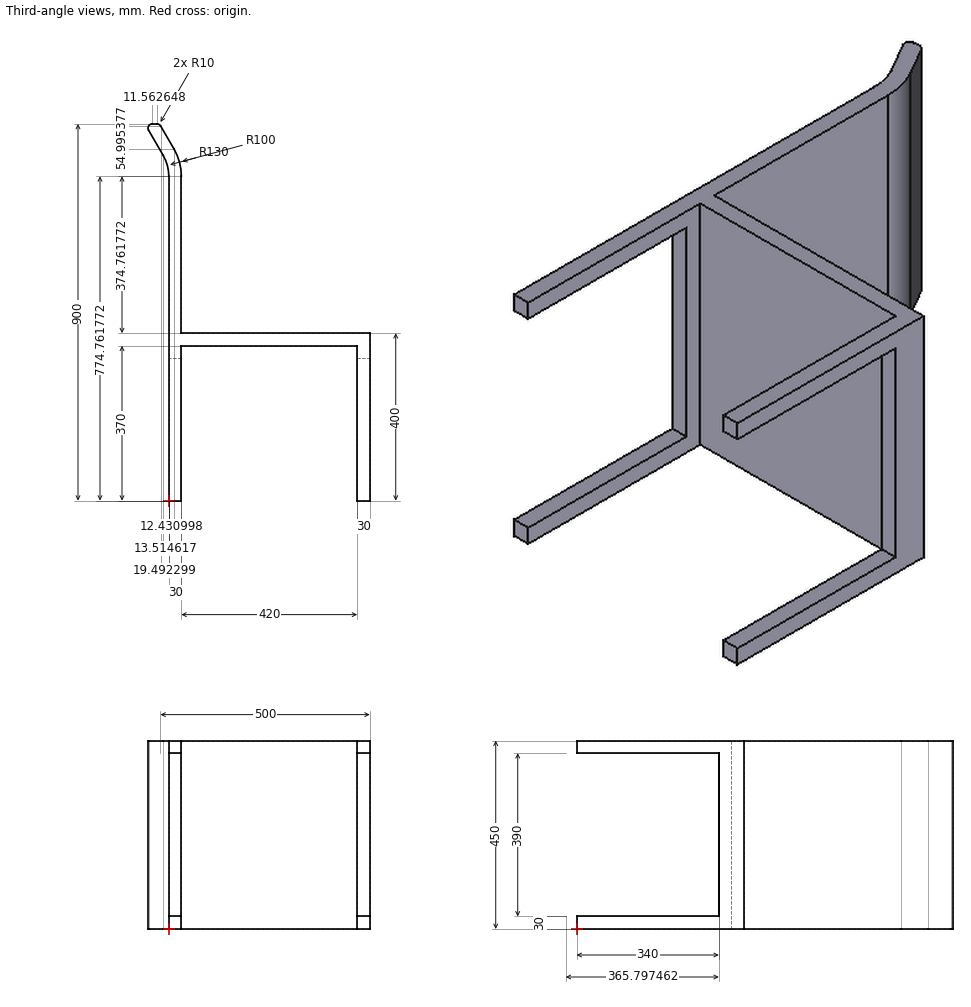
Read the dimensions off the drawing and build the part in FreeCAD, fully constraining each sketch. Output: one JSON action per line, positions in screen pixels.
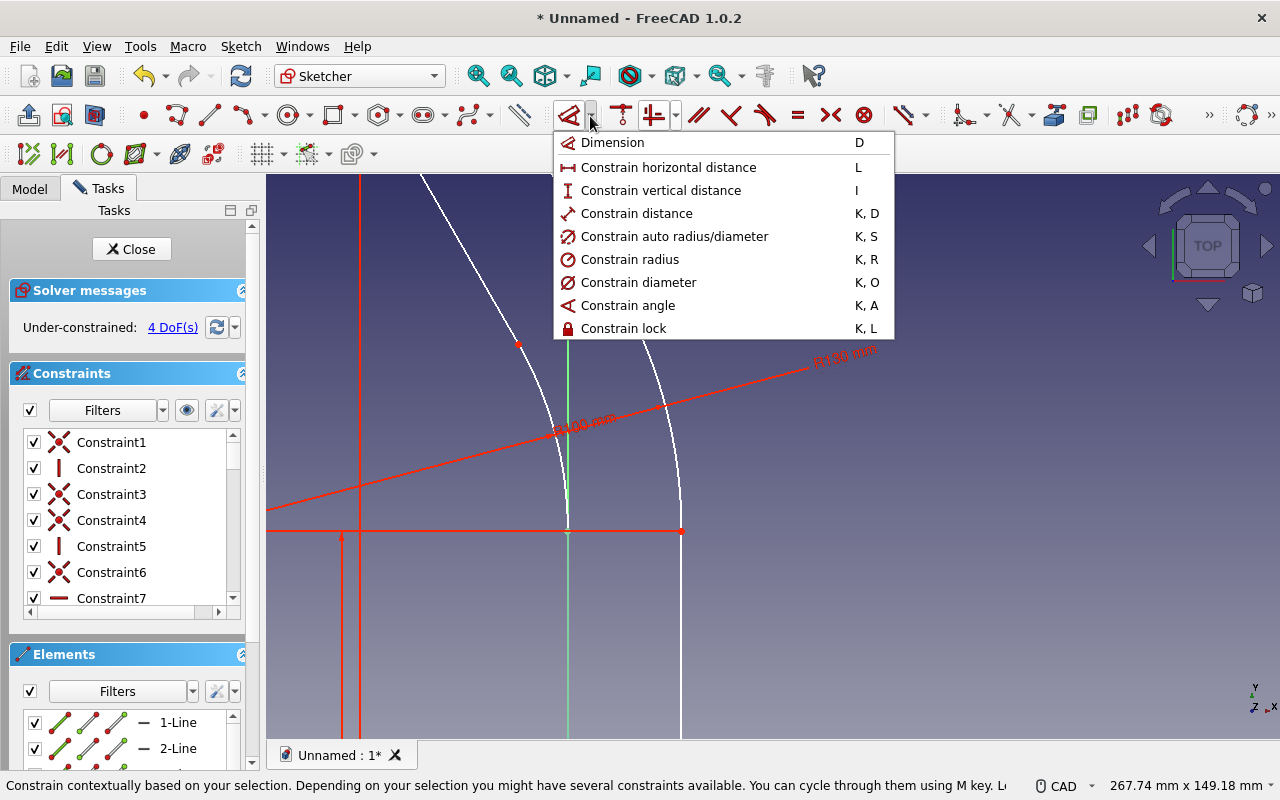
{"action": "left_click", "coordinate": [724, 168]}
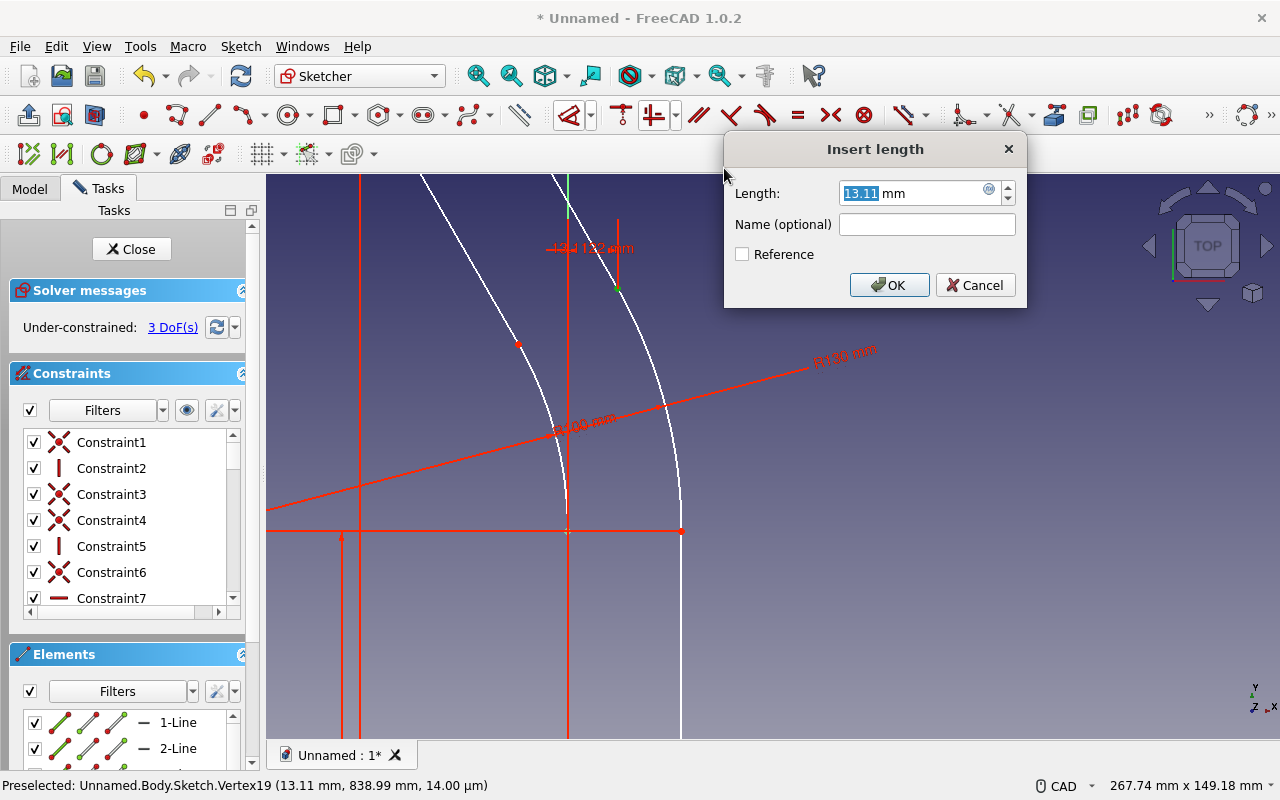
{"action": "type", "text": "12.430998"}
{"action": "key", "text": "Return"}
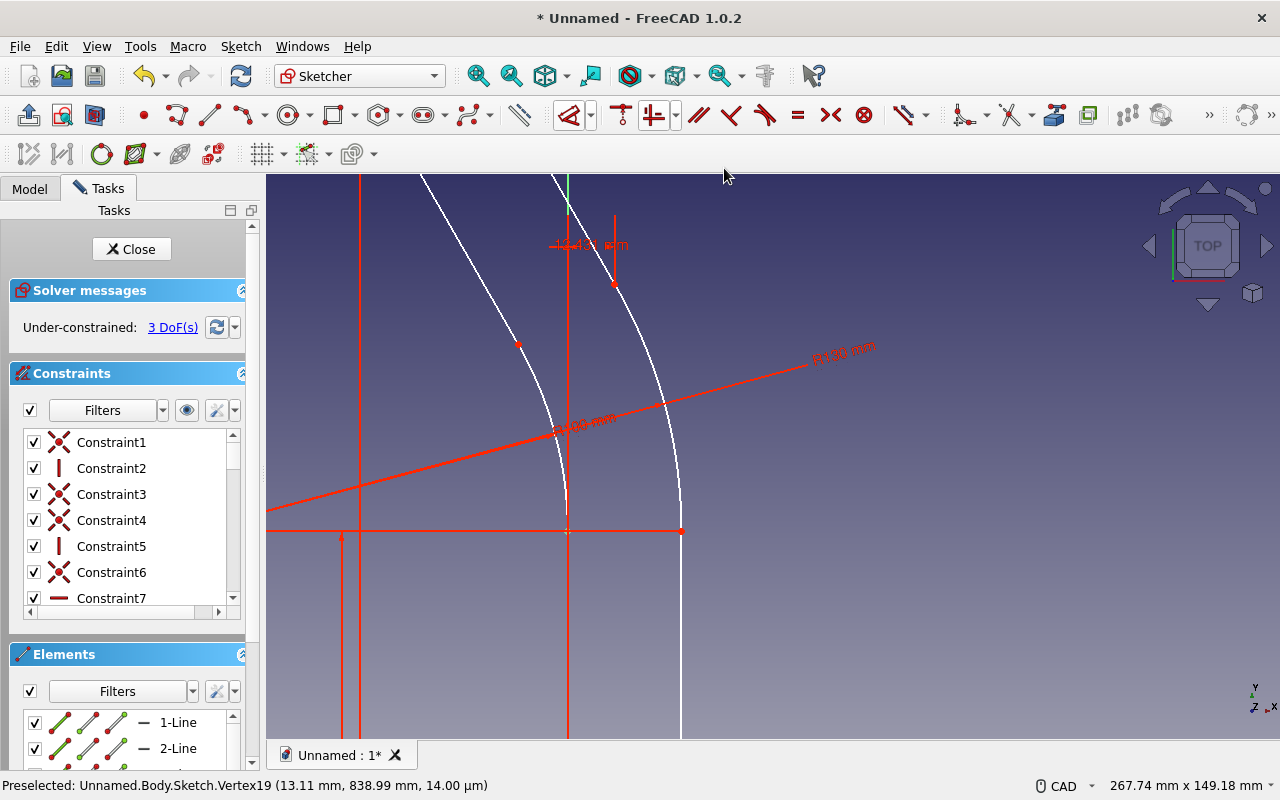
{"action": "scroll", "coordinate": [620, 294], "scroll_direction": "down", "scroll_amount": 11}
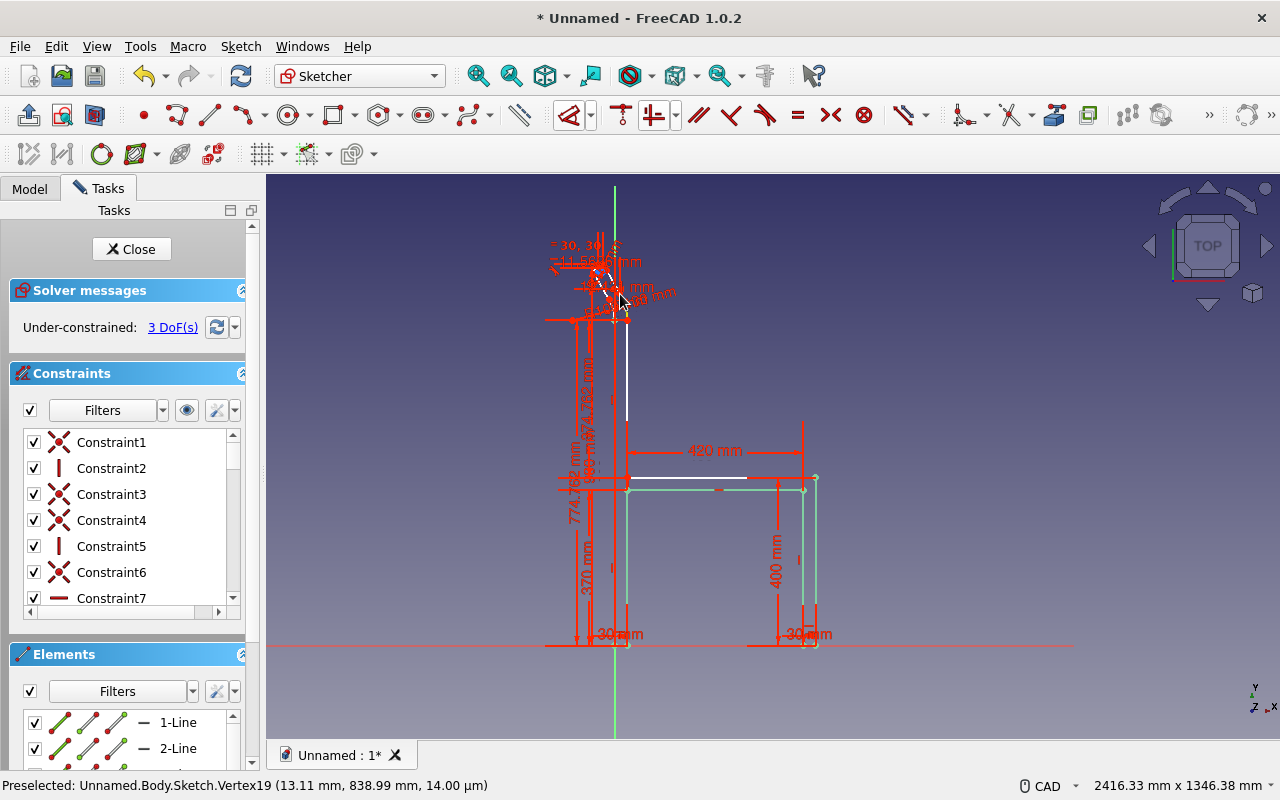
{"action": "scroll", "coordinate": [606, 270], "scroll_direction": "up", "scroll_amount": 8}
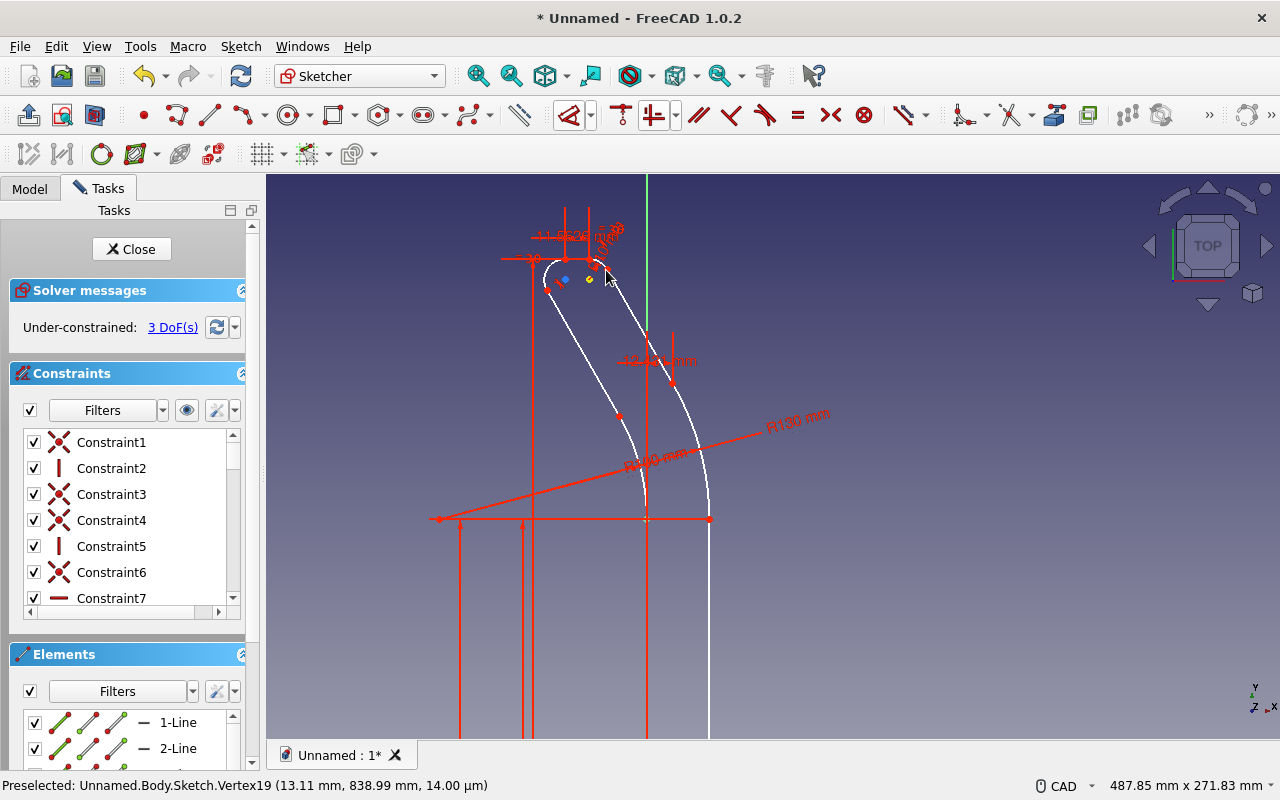
{"action": "left_click", "coordinate": [607, 270]}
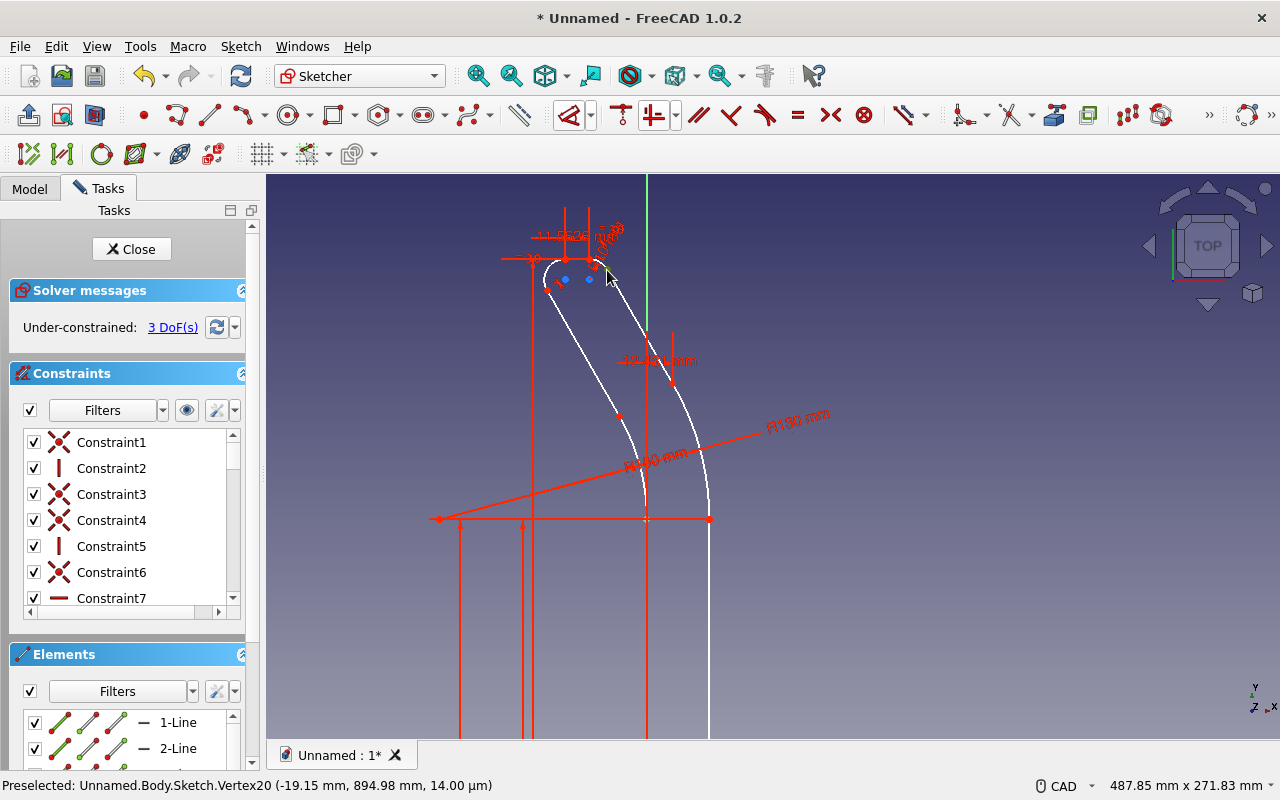
{"action": "left_click", "coordinate": [590, 116]}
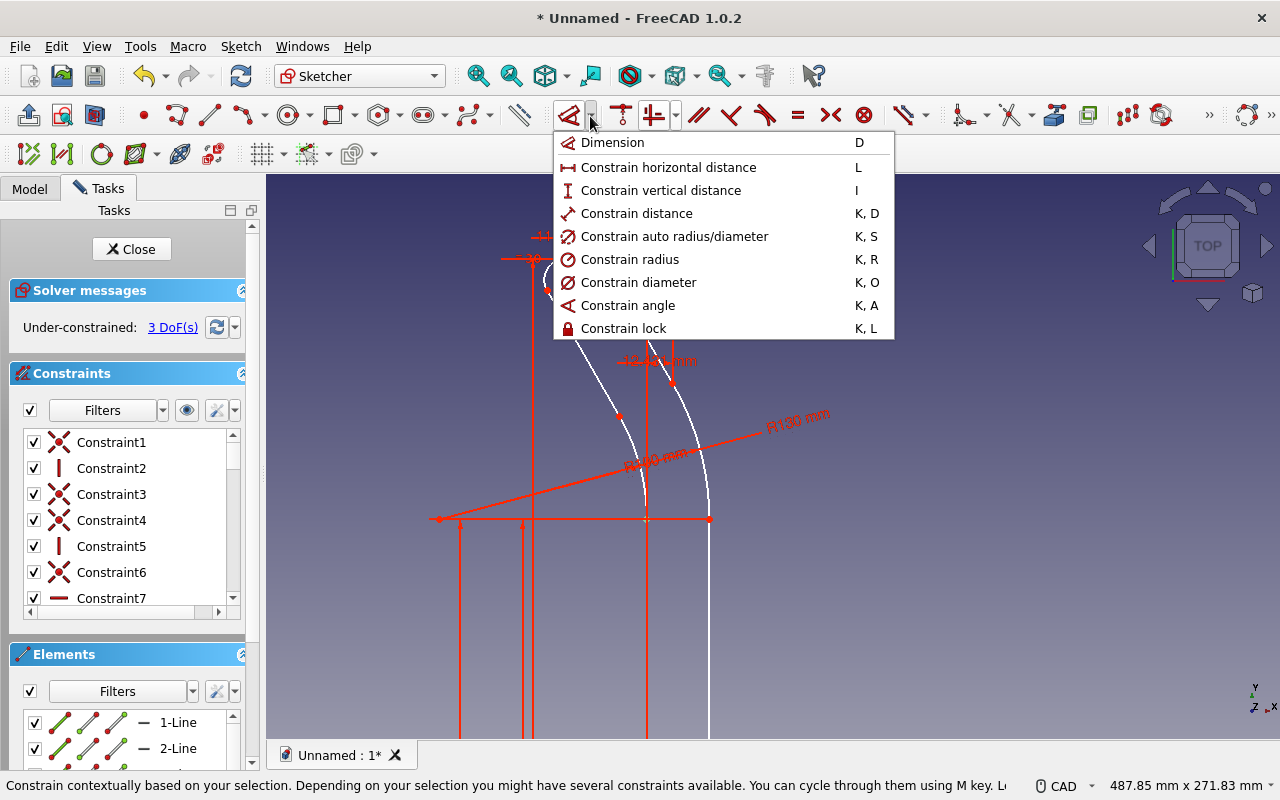
{"action": "left_click", "coordinate": [724, 168]}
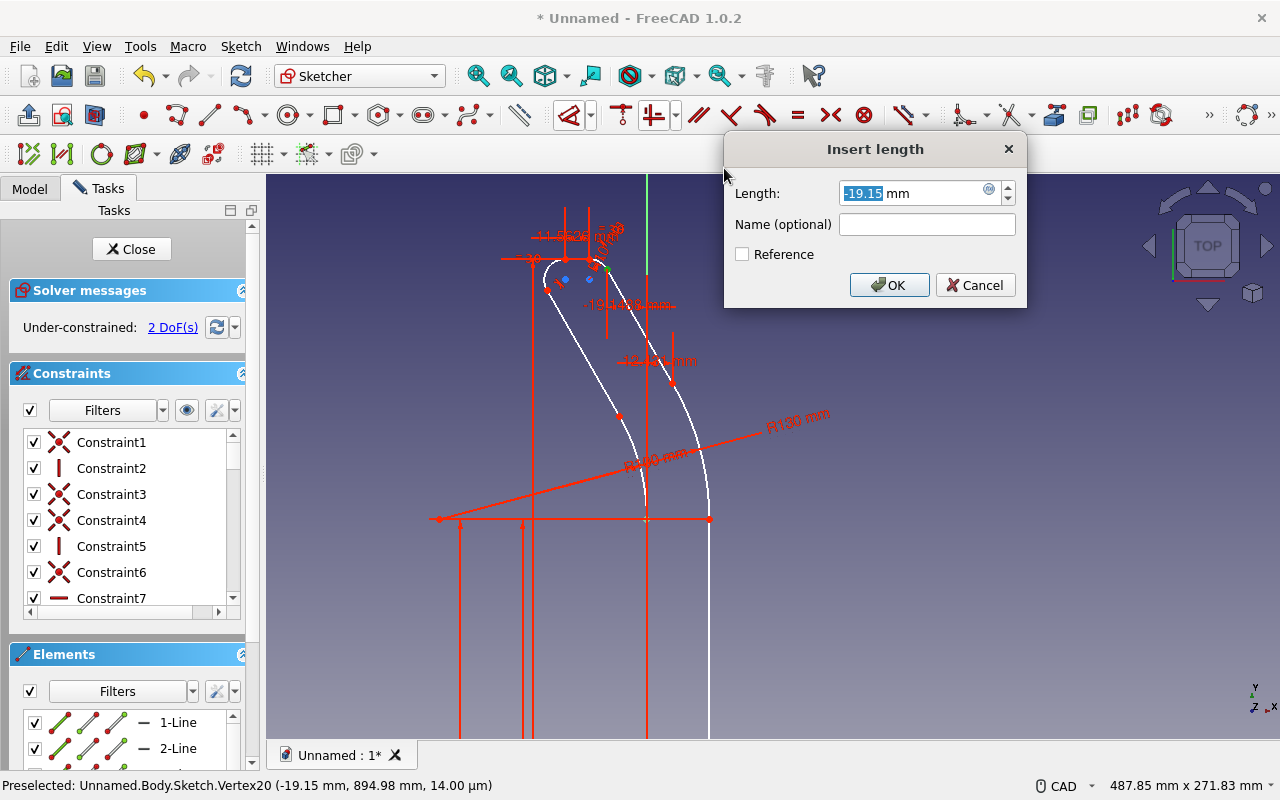
{"action": "type", "text": "-19.492299"}
{"action": "key", "text": "Return"}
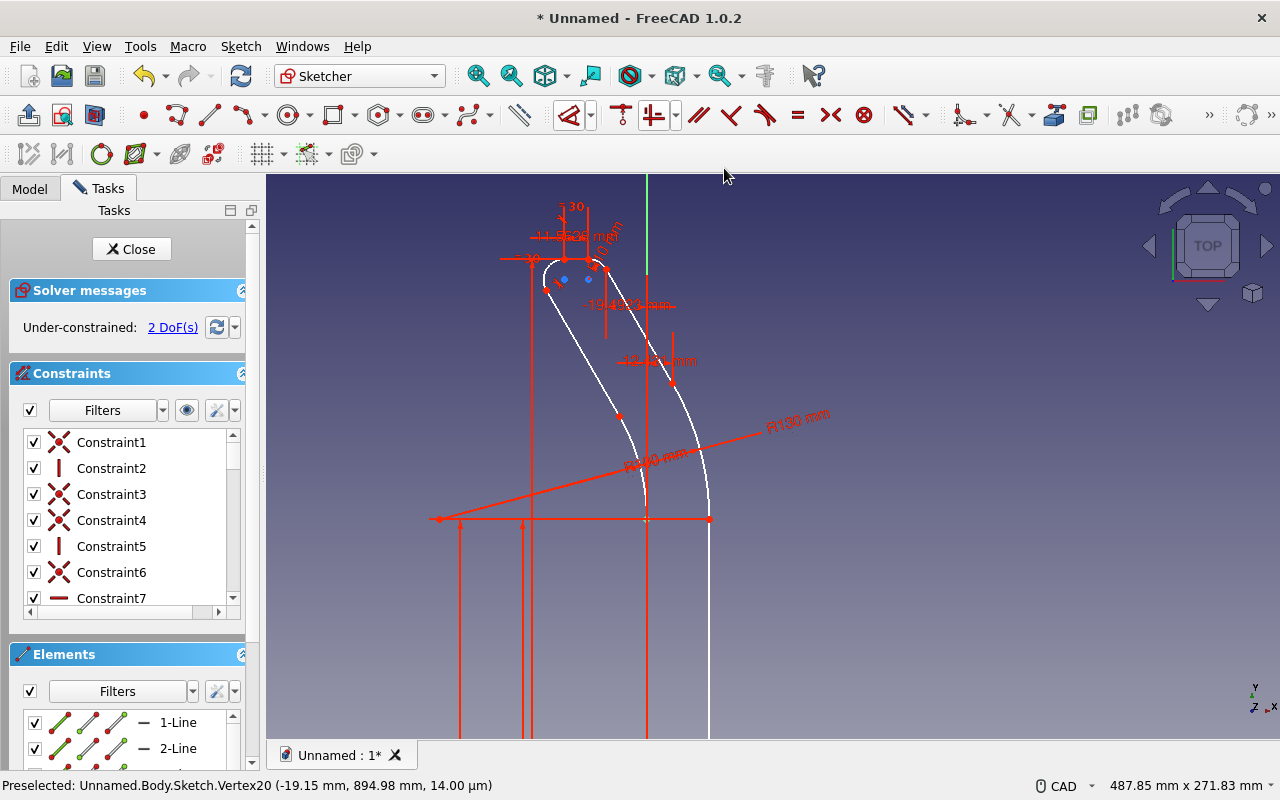
{"action": "scroll", "coordinate": [620, 417], "scroll_direction": "up", "scroll_amount": 2}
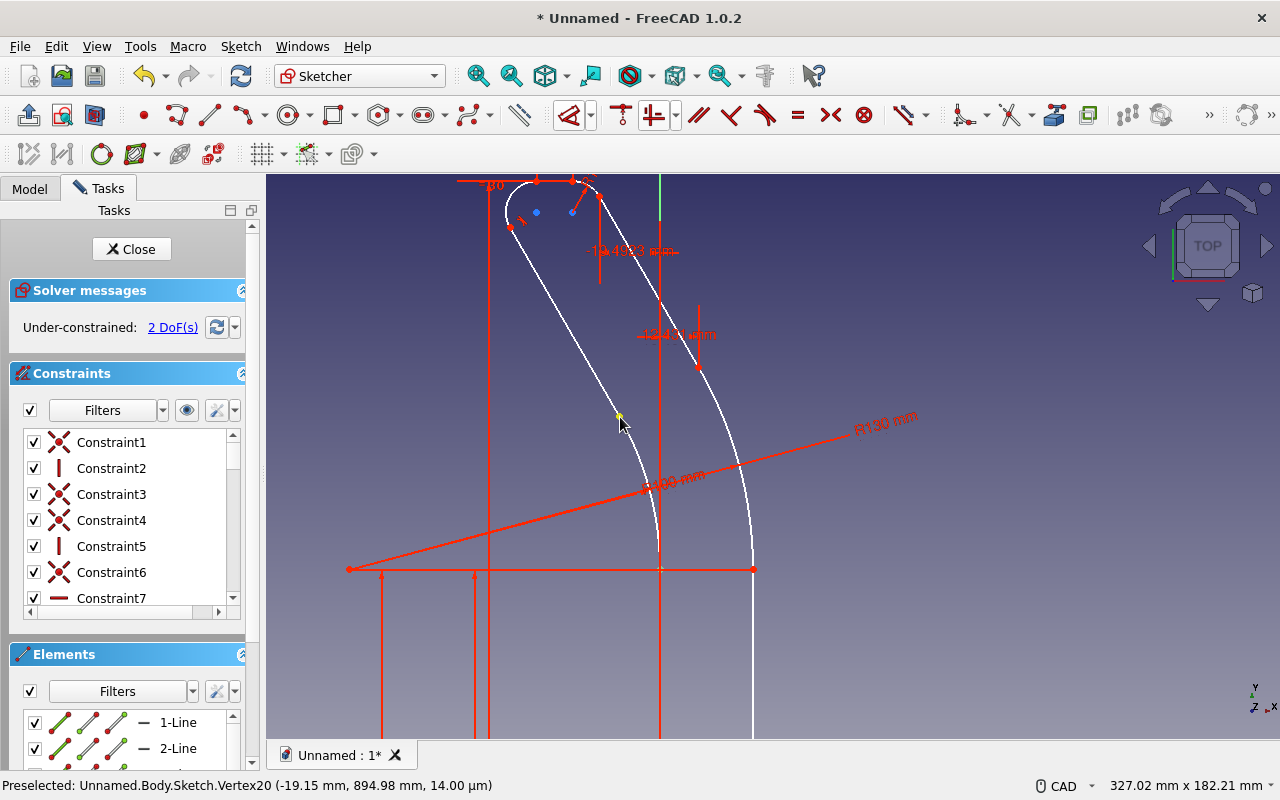
{"action": "left_click", "coordinate": [619, 416]}